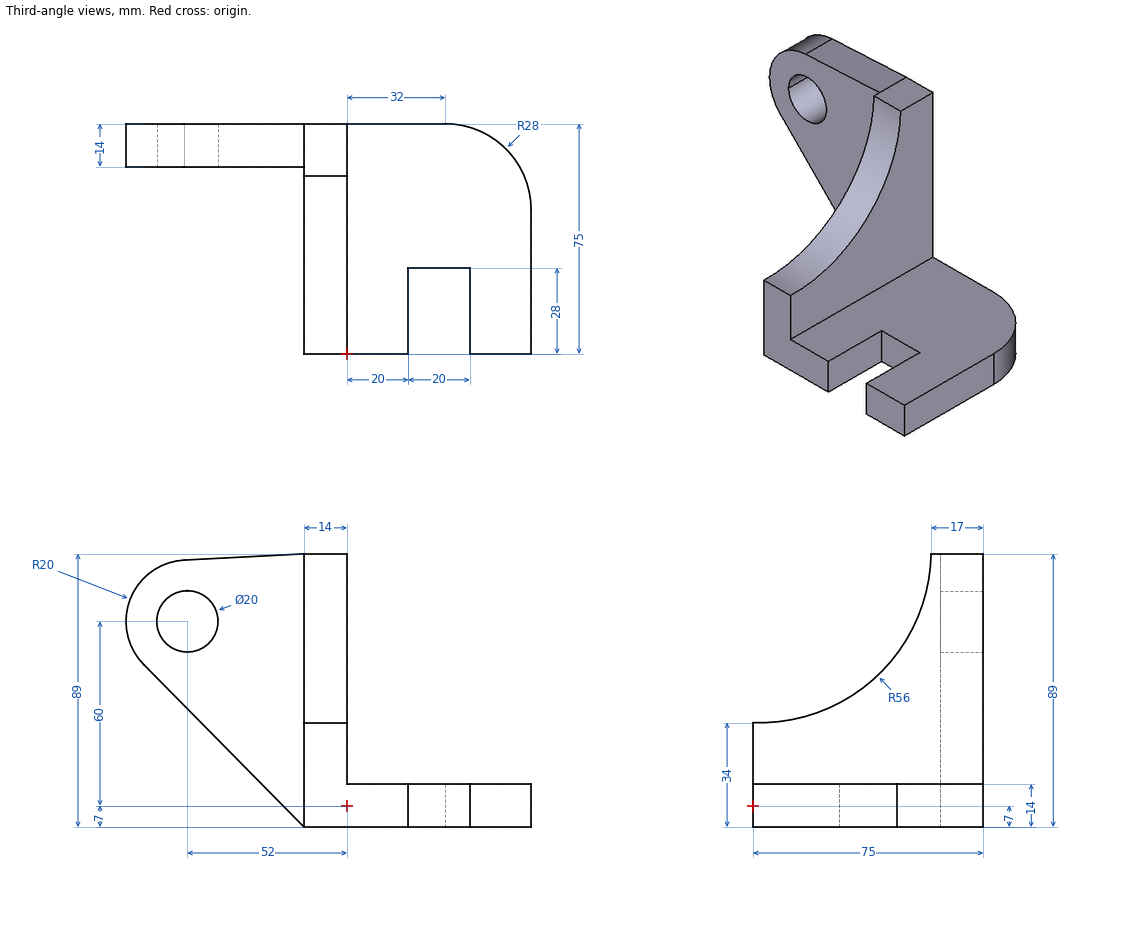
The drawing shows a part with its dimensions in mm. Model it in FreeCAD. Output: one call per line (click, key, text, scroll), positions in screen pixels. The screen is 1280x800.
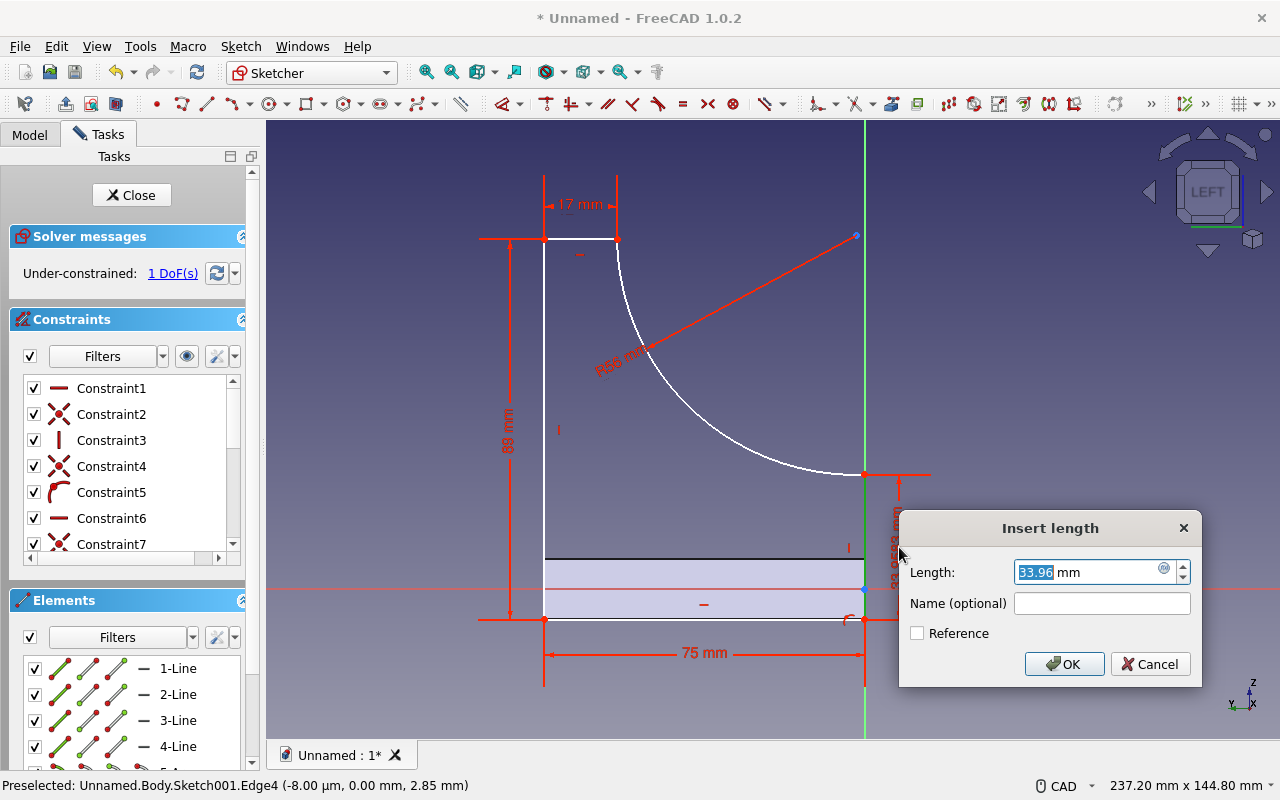
text(34)
key(Return)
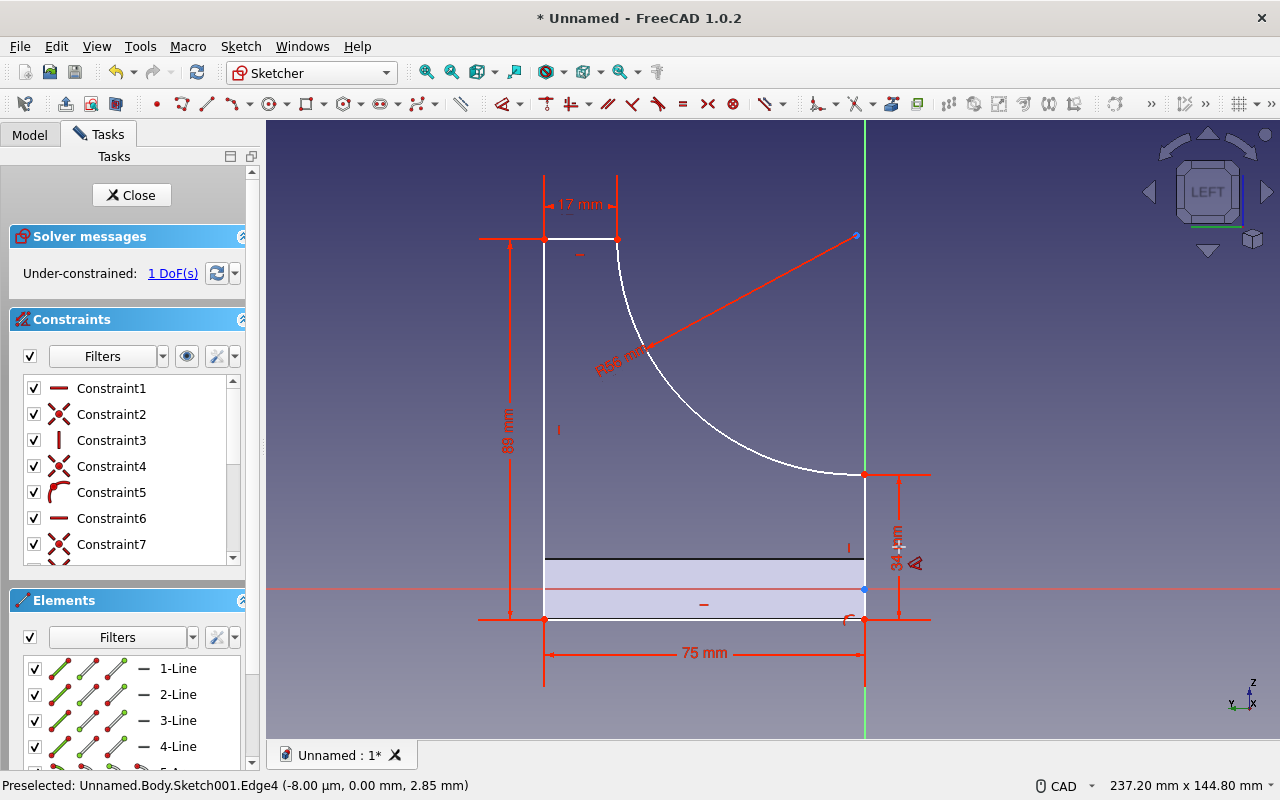
scroll(544, 620, up, 2)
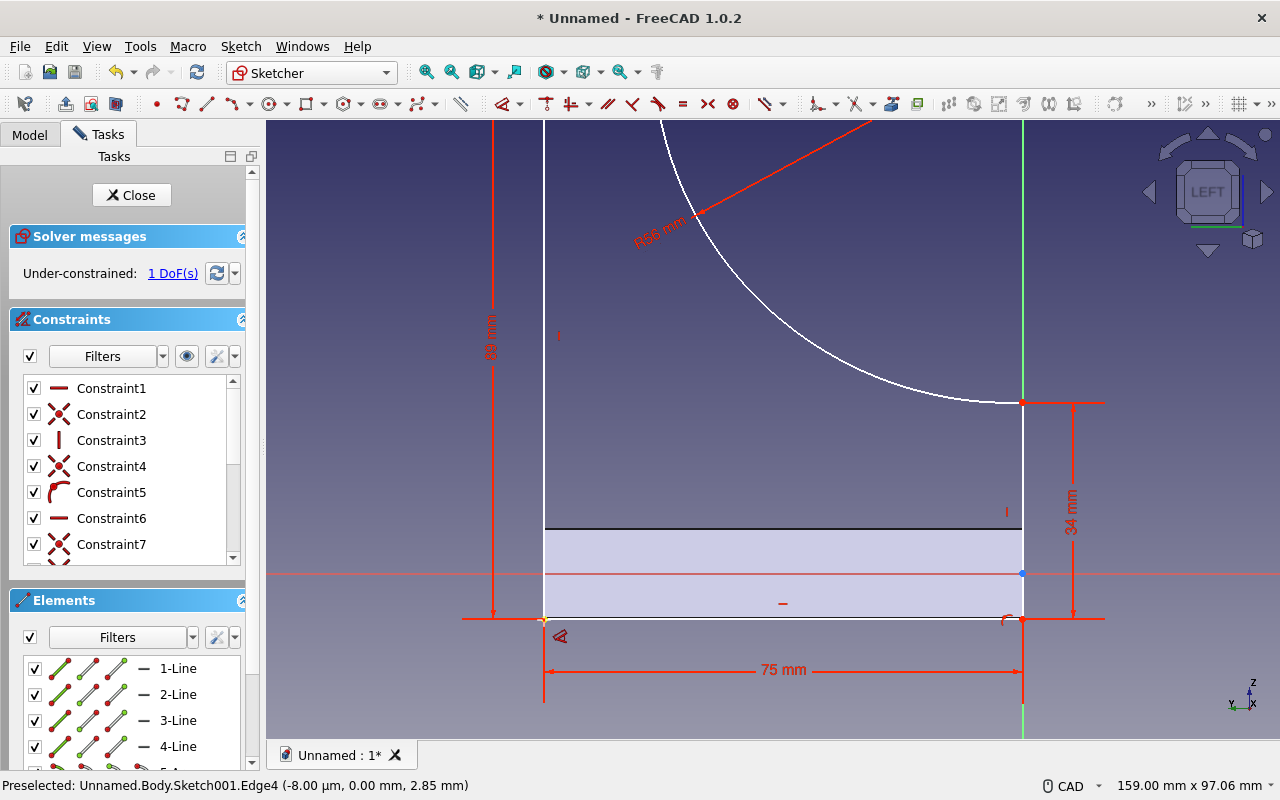
click(544, 619)
click(1057, 597)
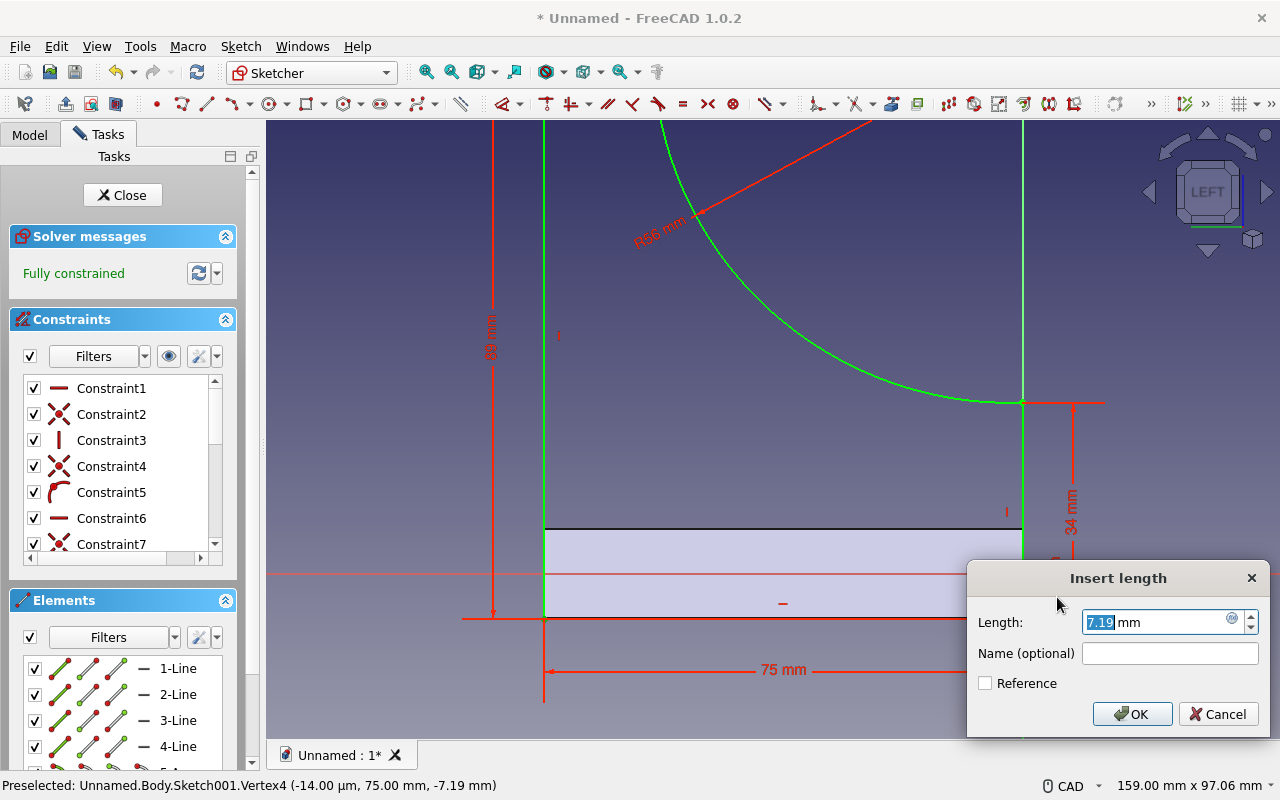
text(7)
key(Return)
key(Escape)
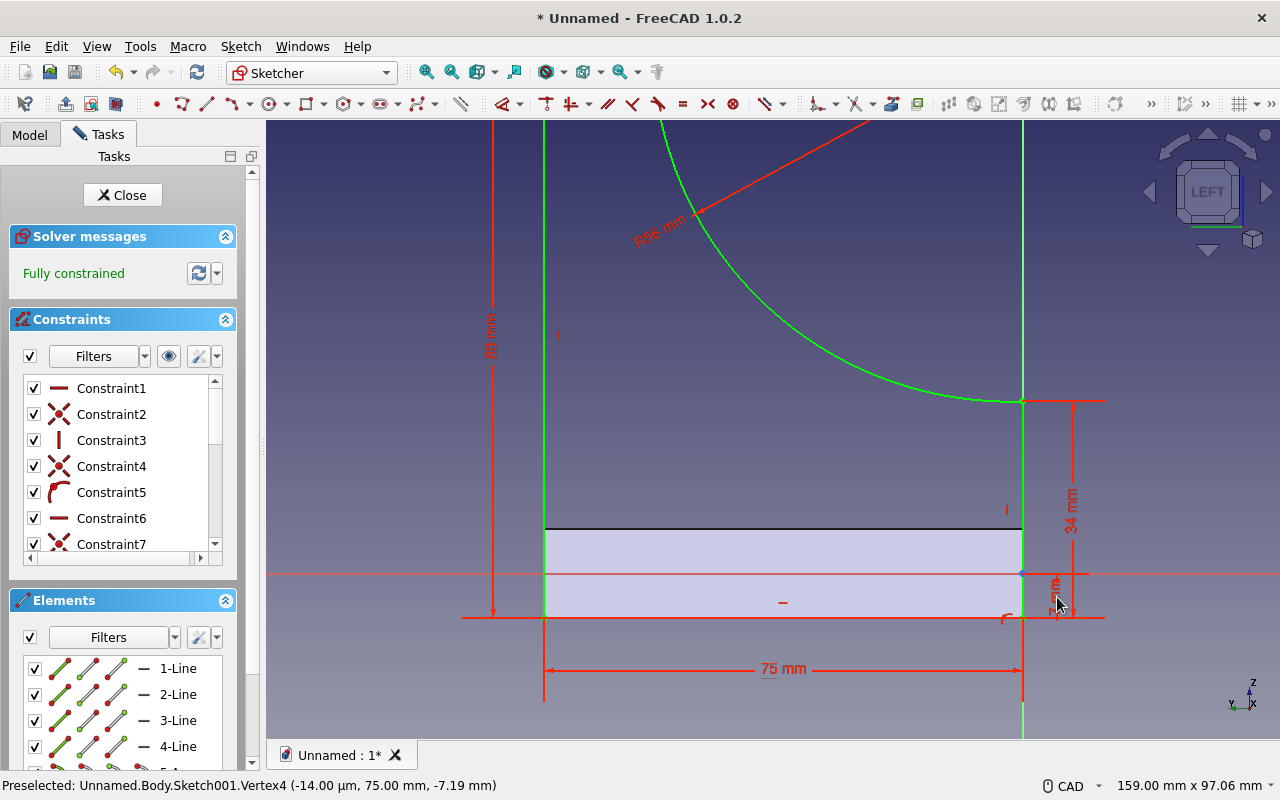
click(123, 195)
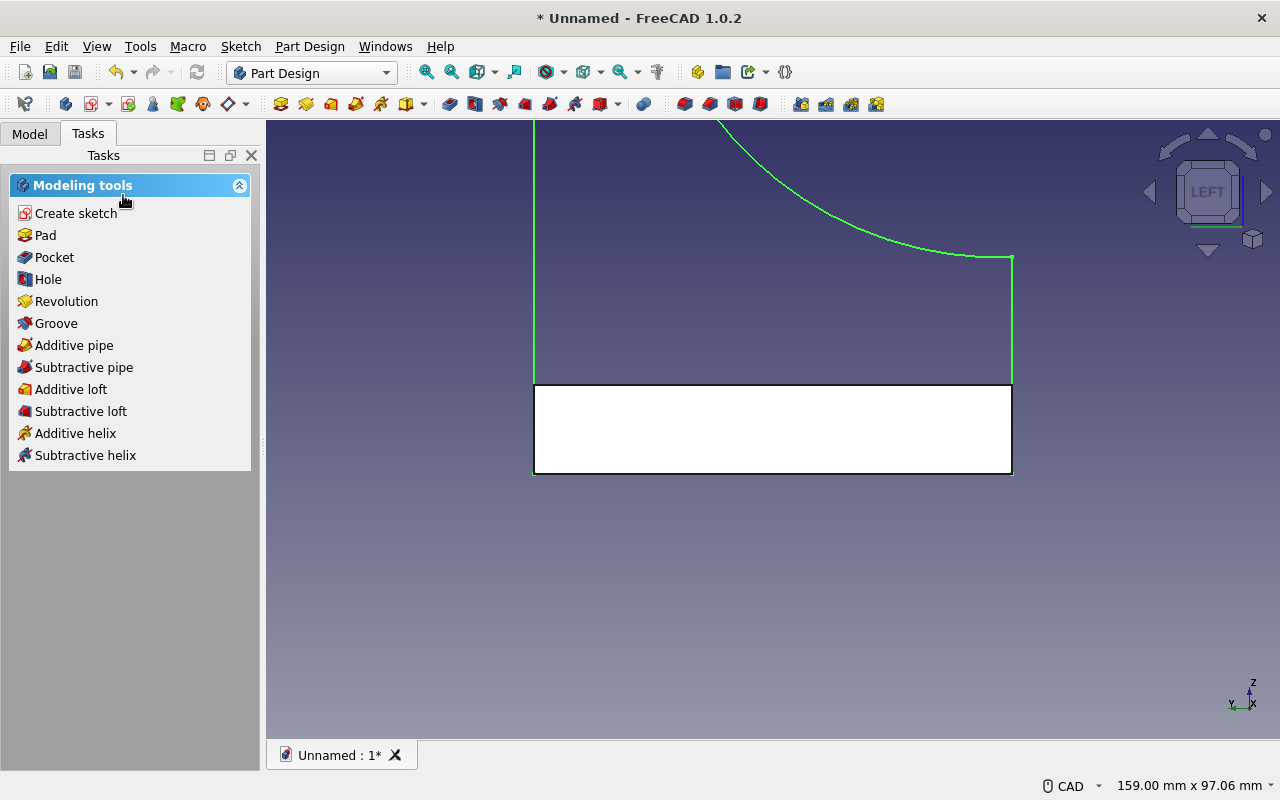
click(281, 104)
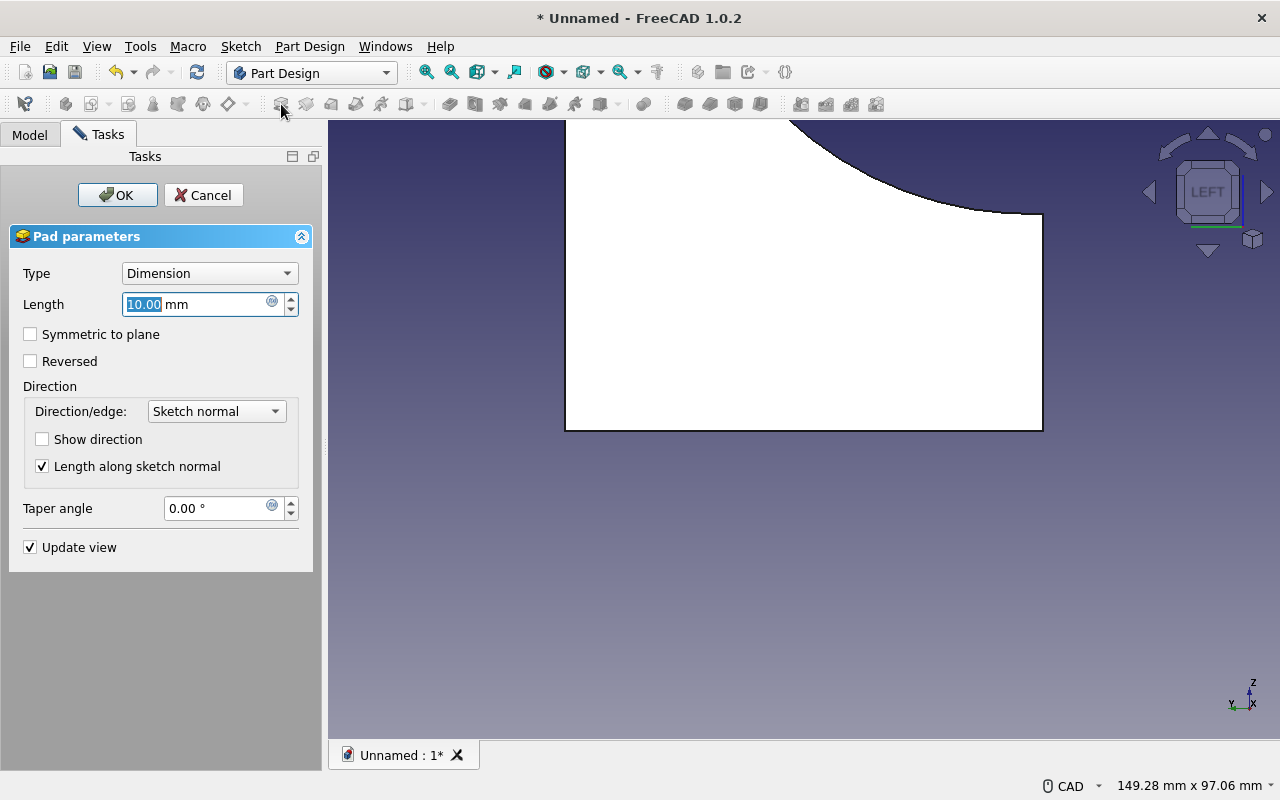
text(14)
key(Tab)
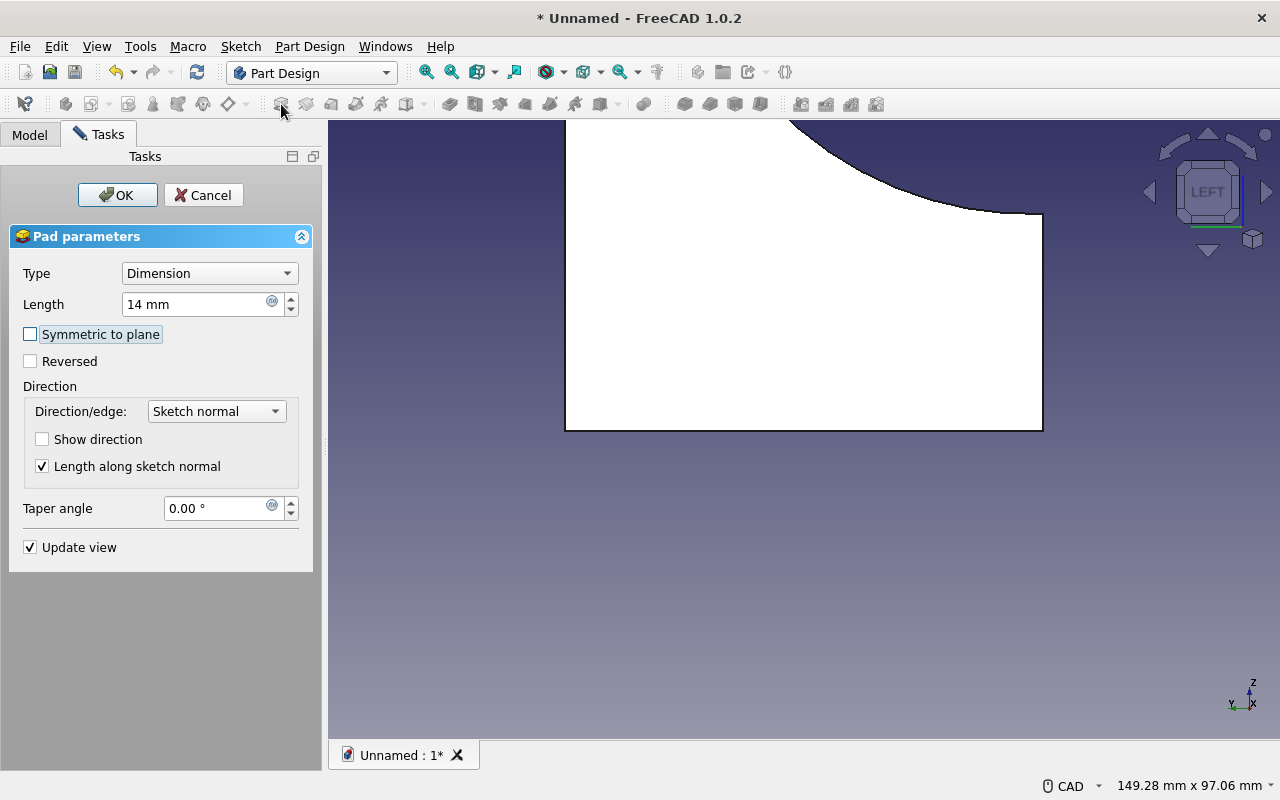
click(118, 195)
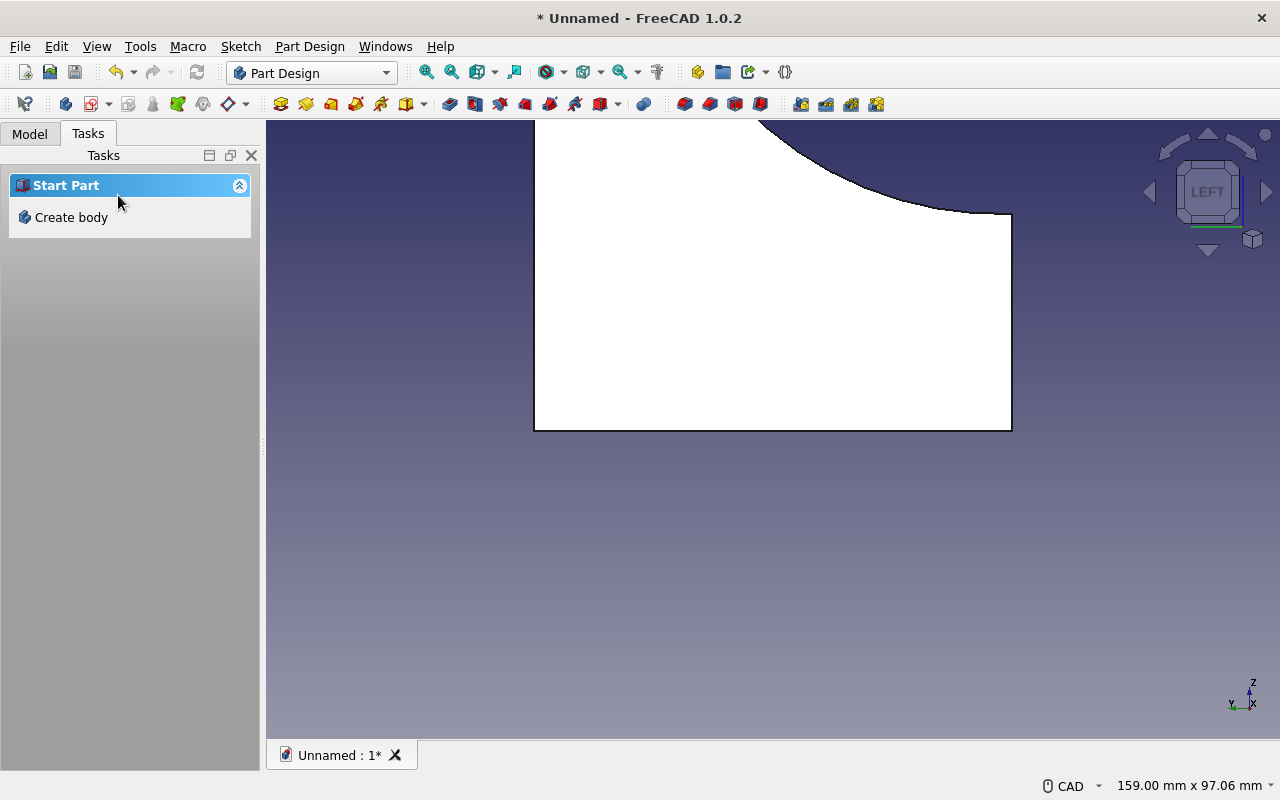
click(427, 72)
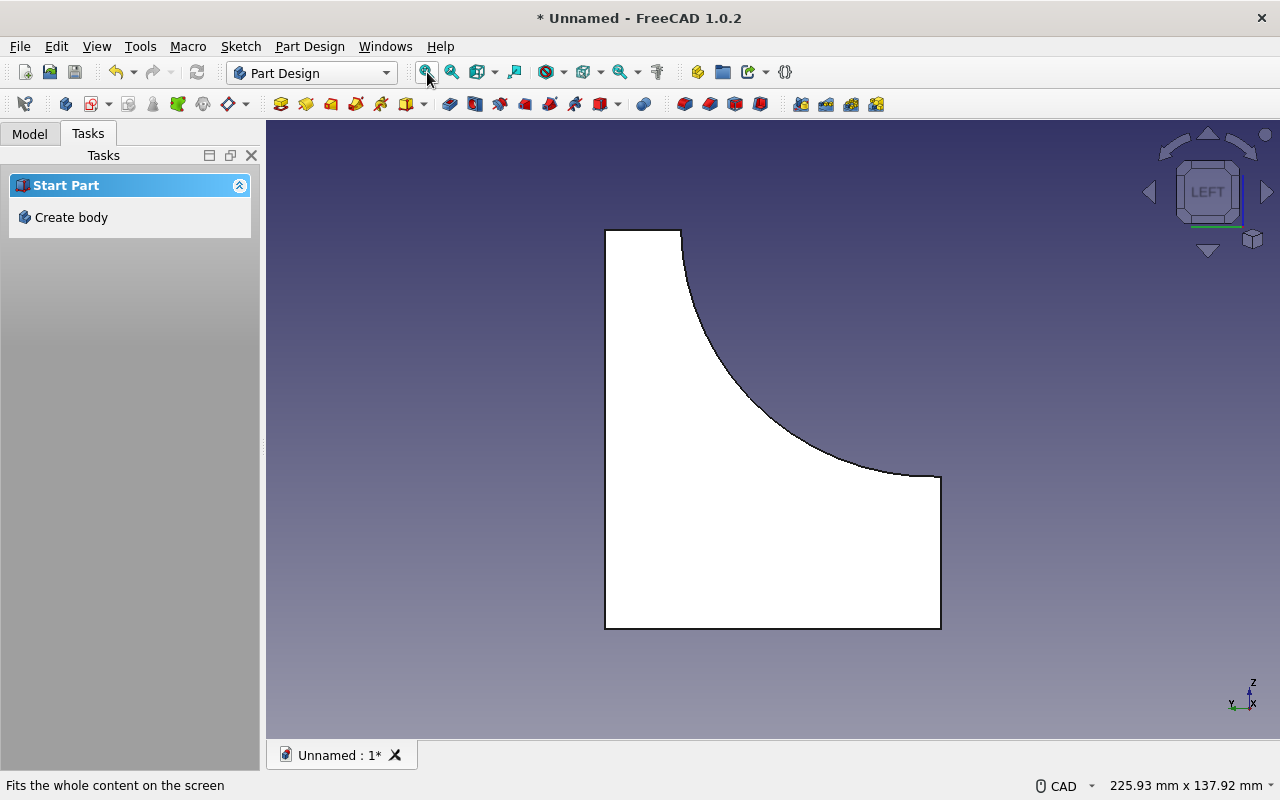
key(4)